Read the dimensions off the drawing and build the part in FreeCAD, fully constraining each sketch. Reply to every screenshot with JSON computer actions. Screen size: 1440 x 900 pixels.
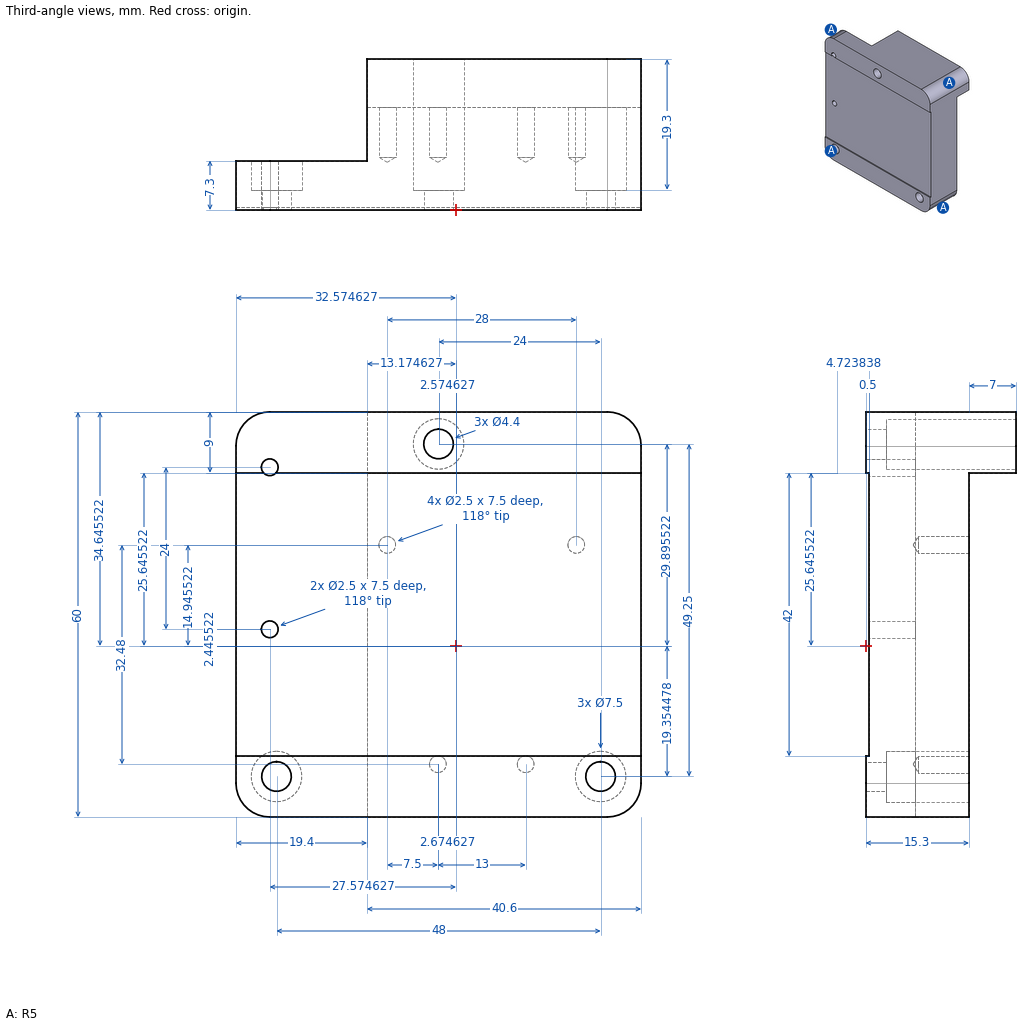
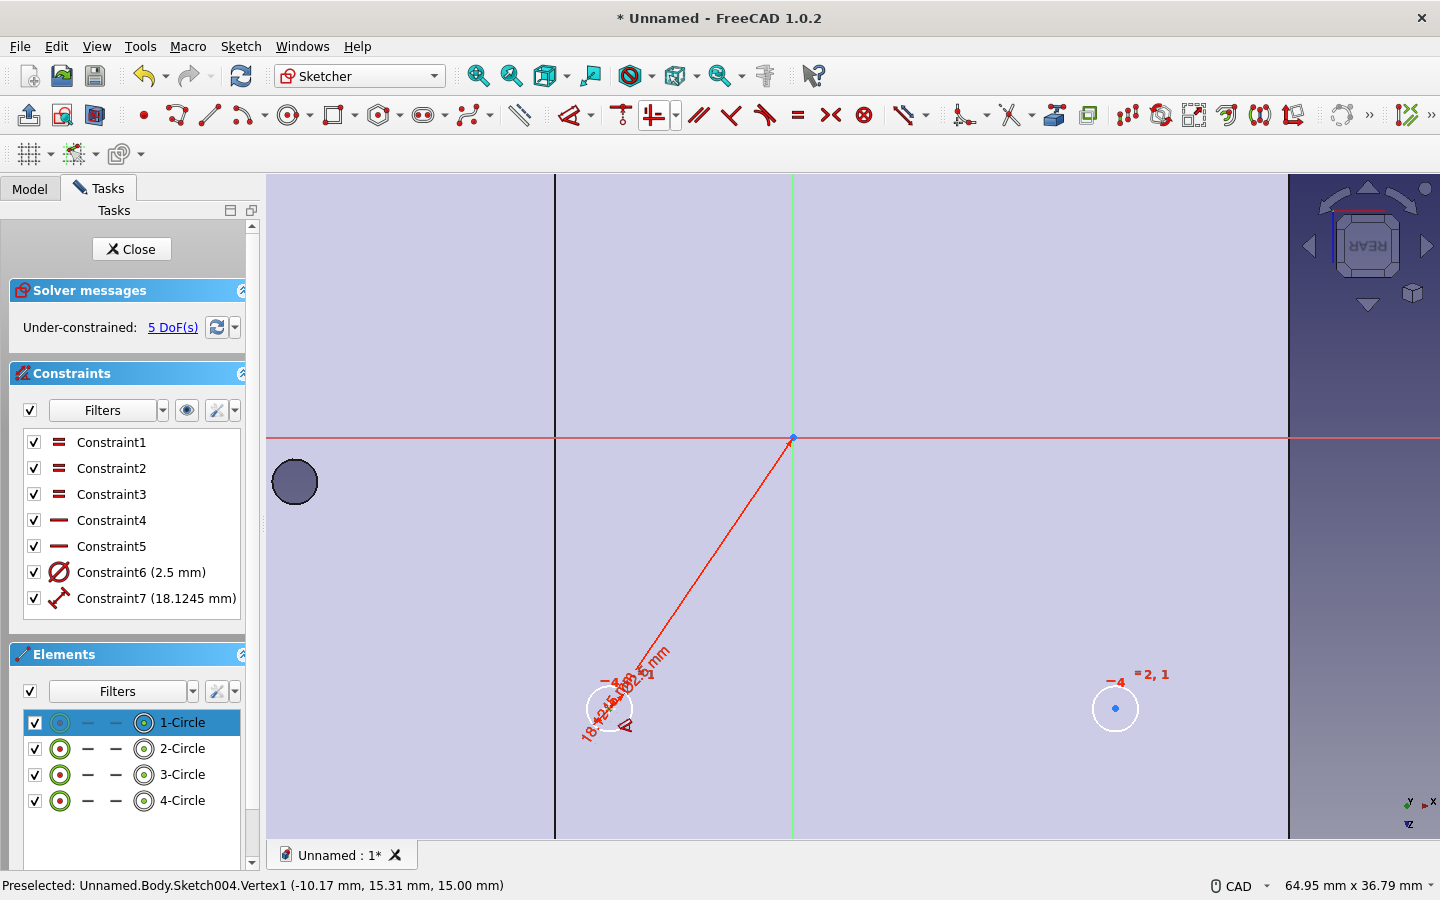
{"action": "left_click", "coordinate": [1115, 709]}
{"action": "left_click", "coordinate": [862, 743]}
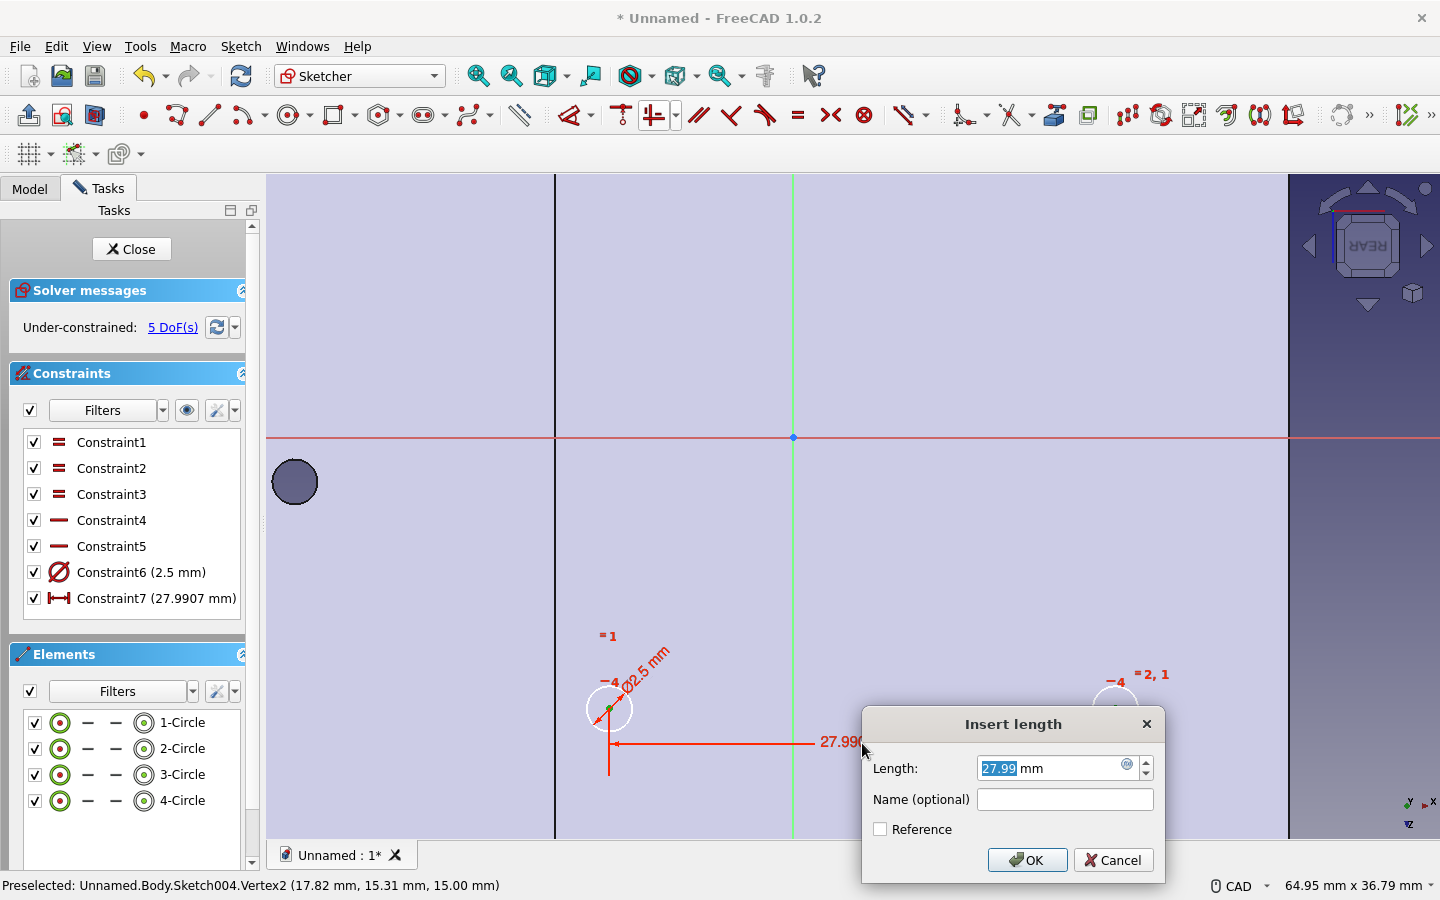
{"action": "type", "text": "28"}
{"action": "key", "text": "Return"}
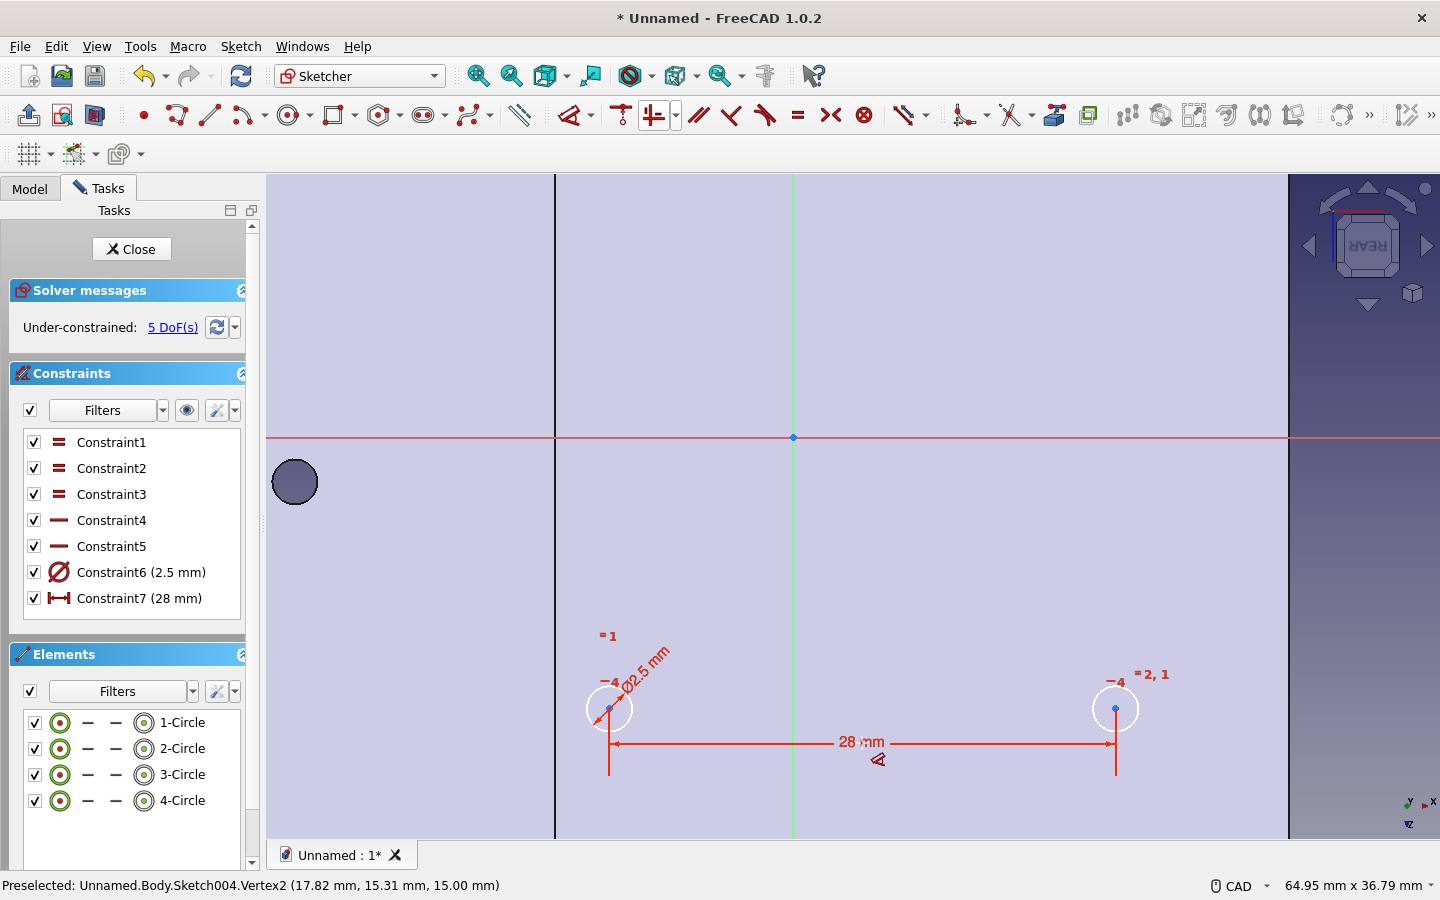
{"action": "scroll", "coordinate": [626, 694], "scroll_direction": "down", "scroll_amount": 2}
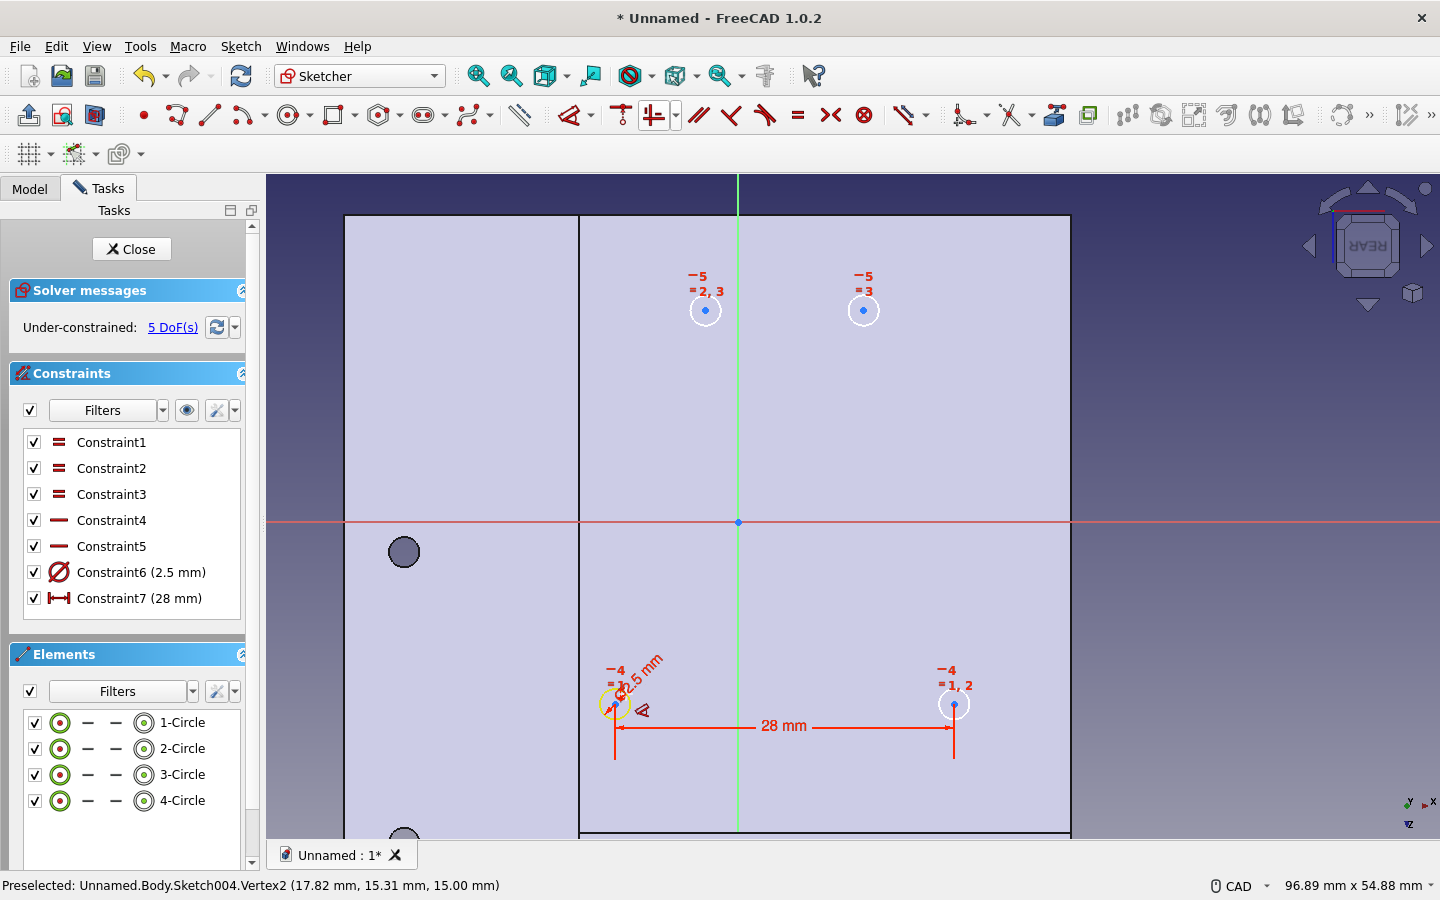
{"action": "left_click", "coordinate": [706, 311]}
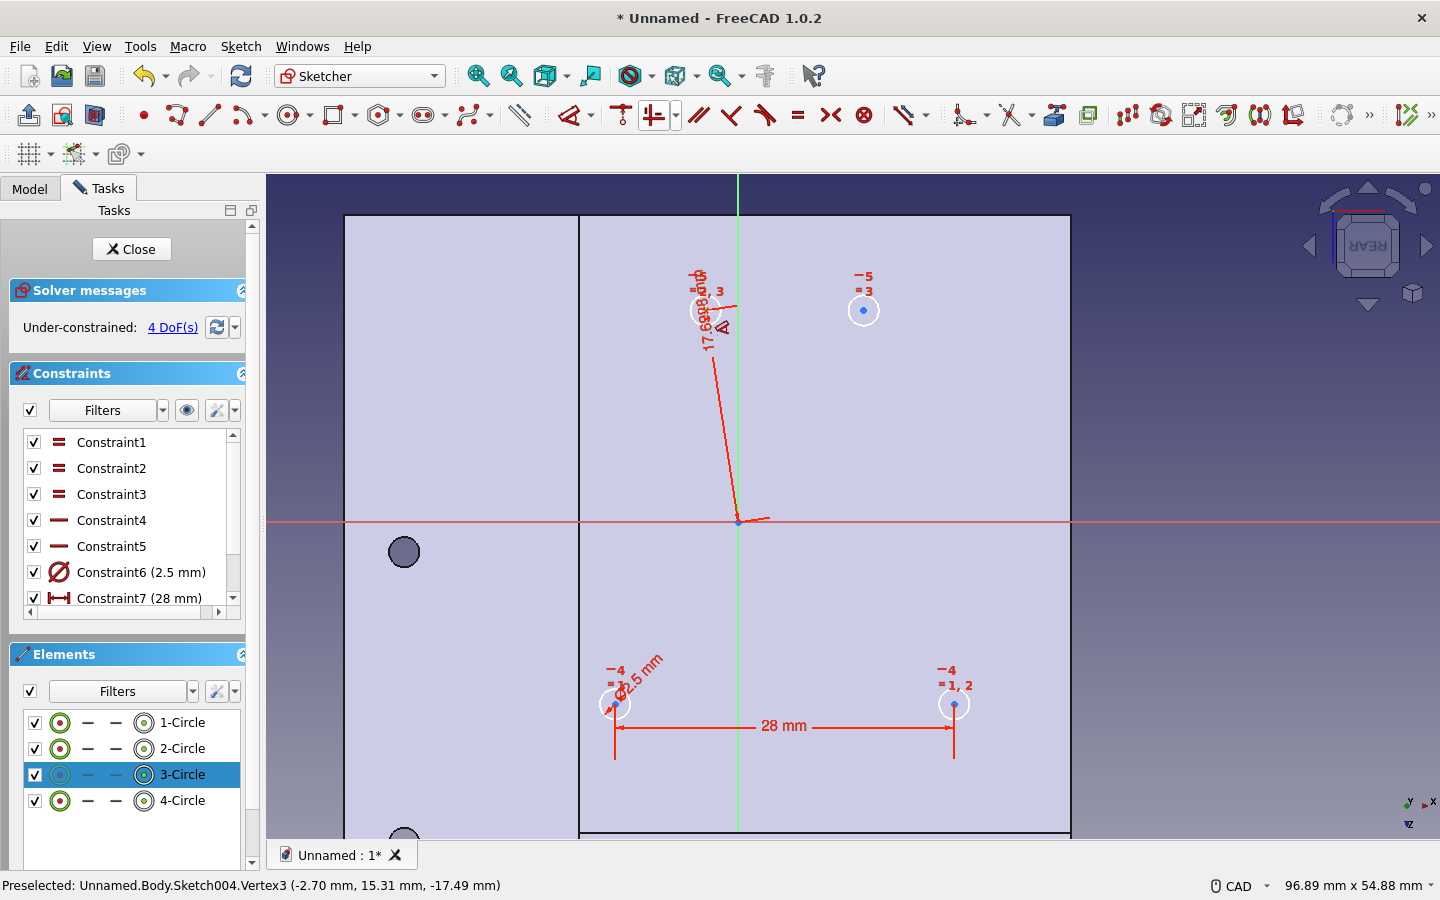
{"action": "left_click", "coordinate": [864, 311]}
{"action": "left_click", "coordinate": [785, 277]}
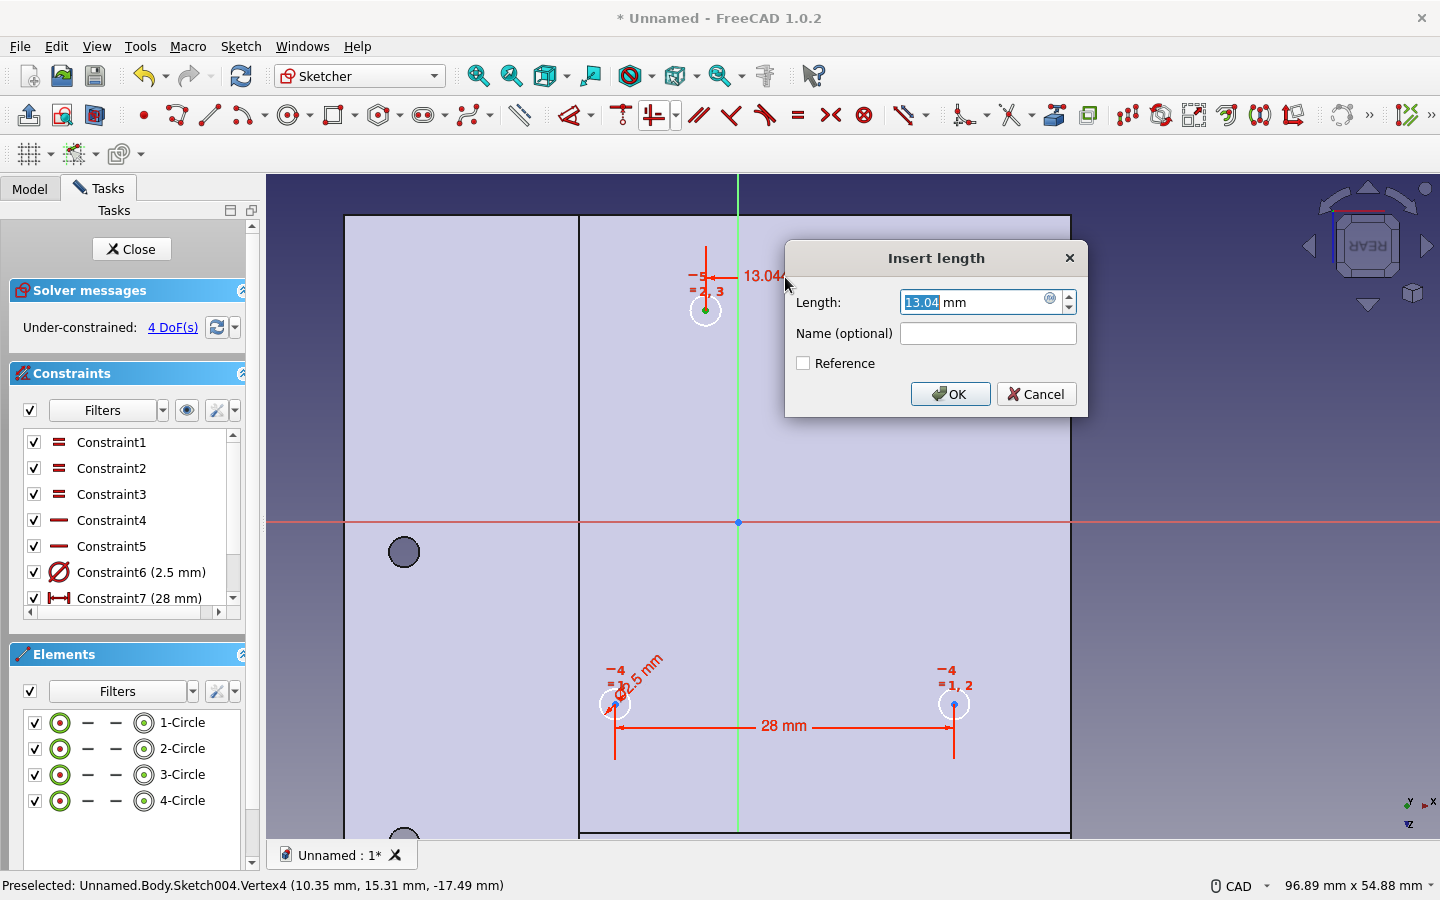
{"action": "type", "text": "13"}
{"action": "key", "text": "Return"}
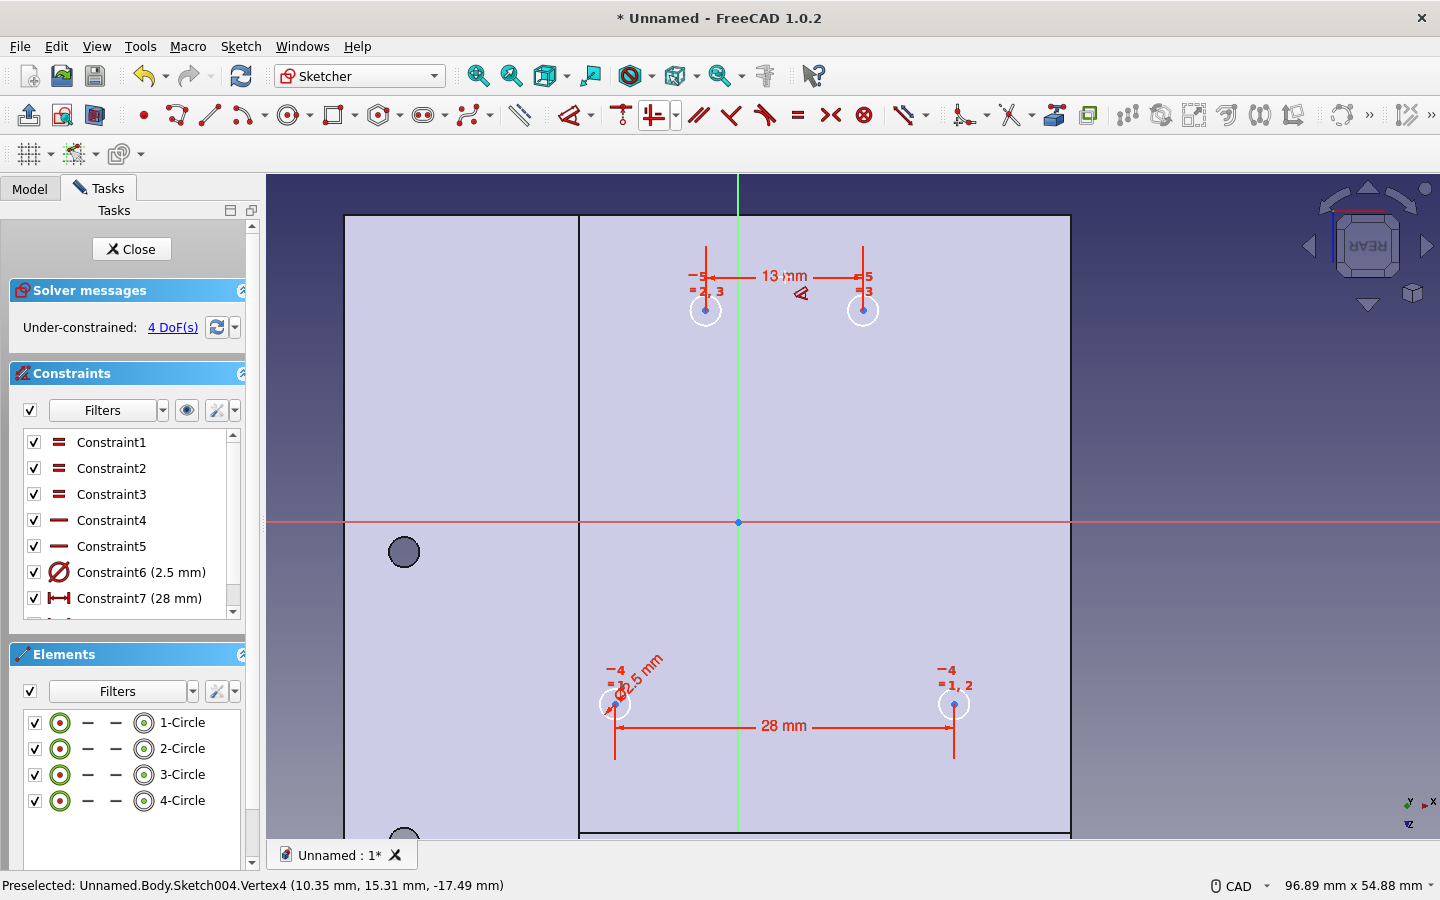
{"action": "left_click", "coordinate": [615, 704]}